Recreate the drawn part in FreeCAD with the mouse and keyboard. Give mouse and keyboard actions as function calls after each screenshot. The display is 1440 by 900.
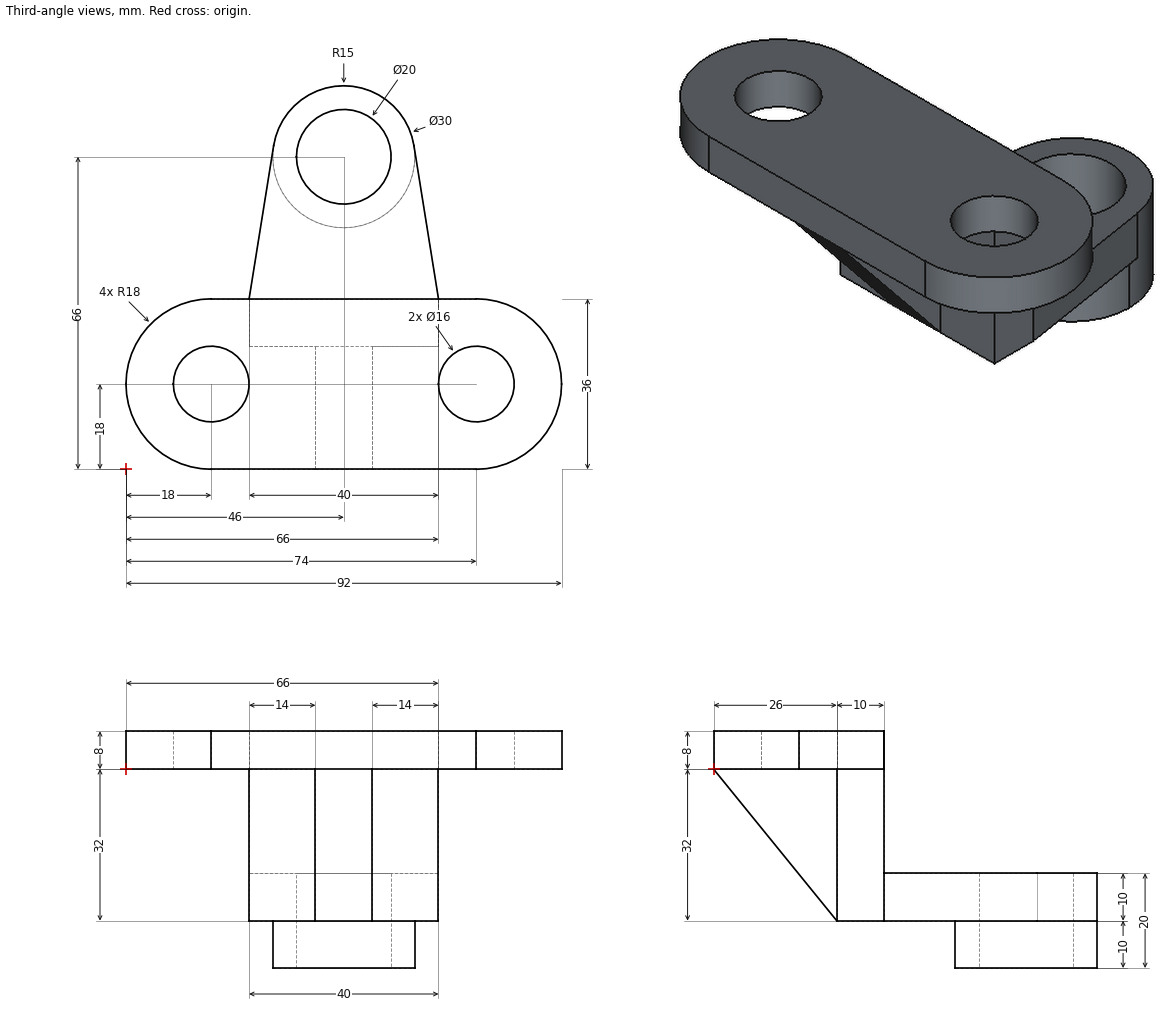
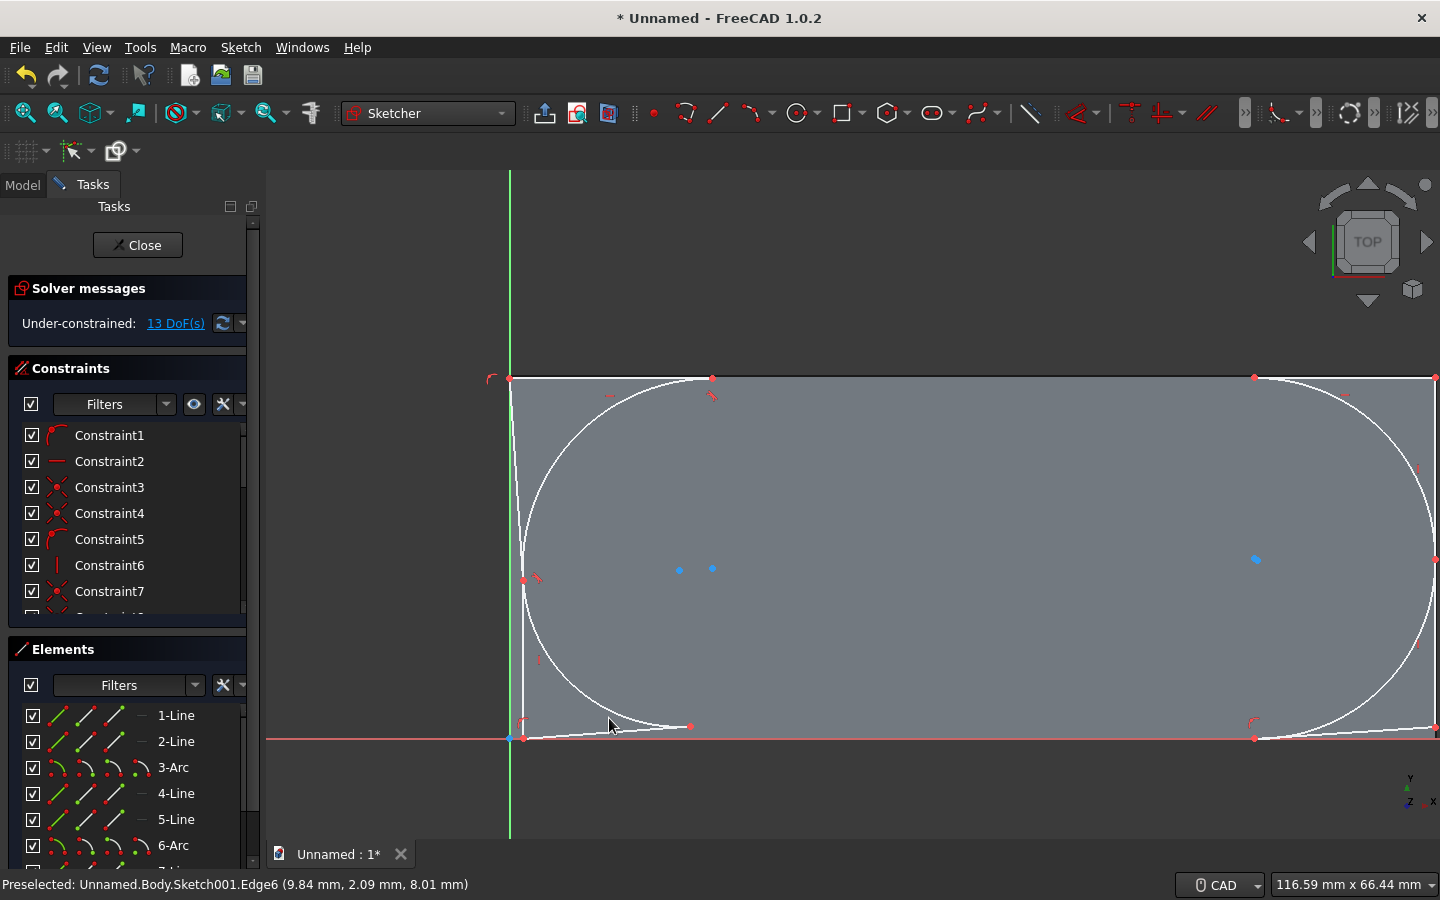
click(573, 735)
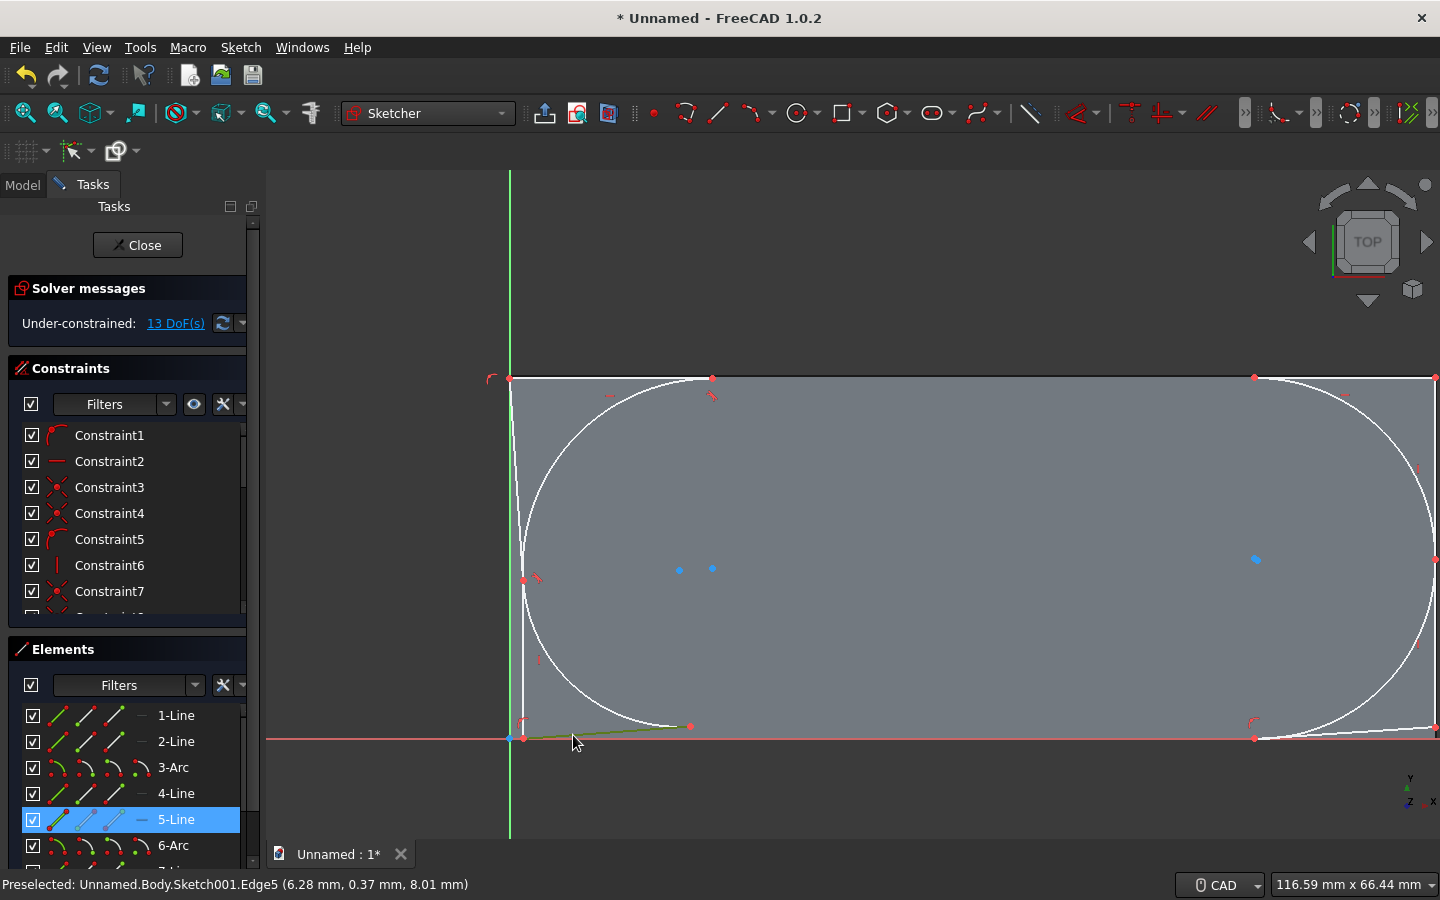
click(545, 651)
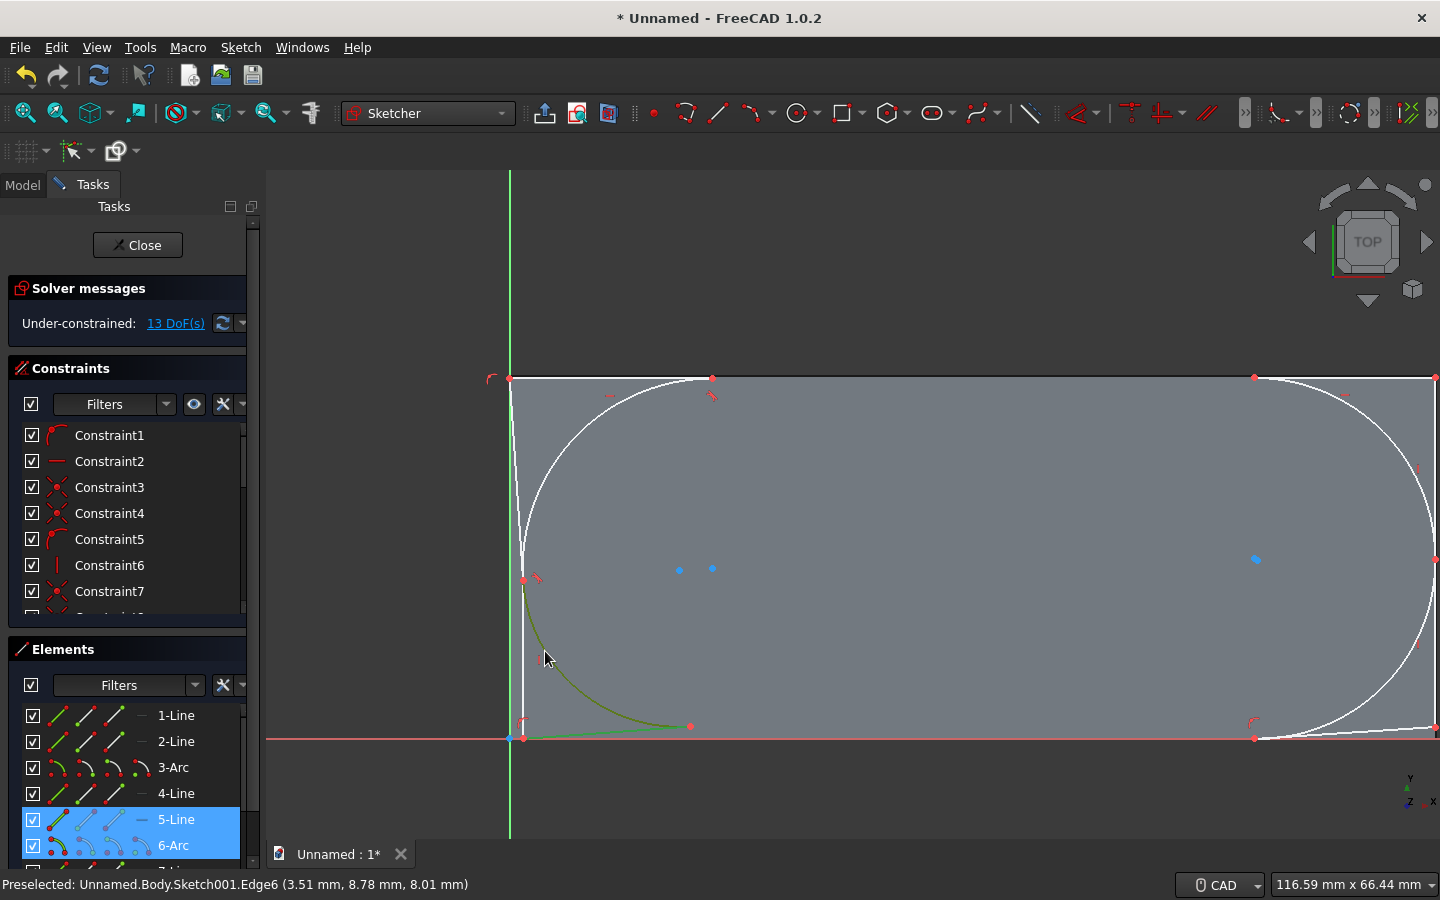
key(t)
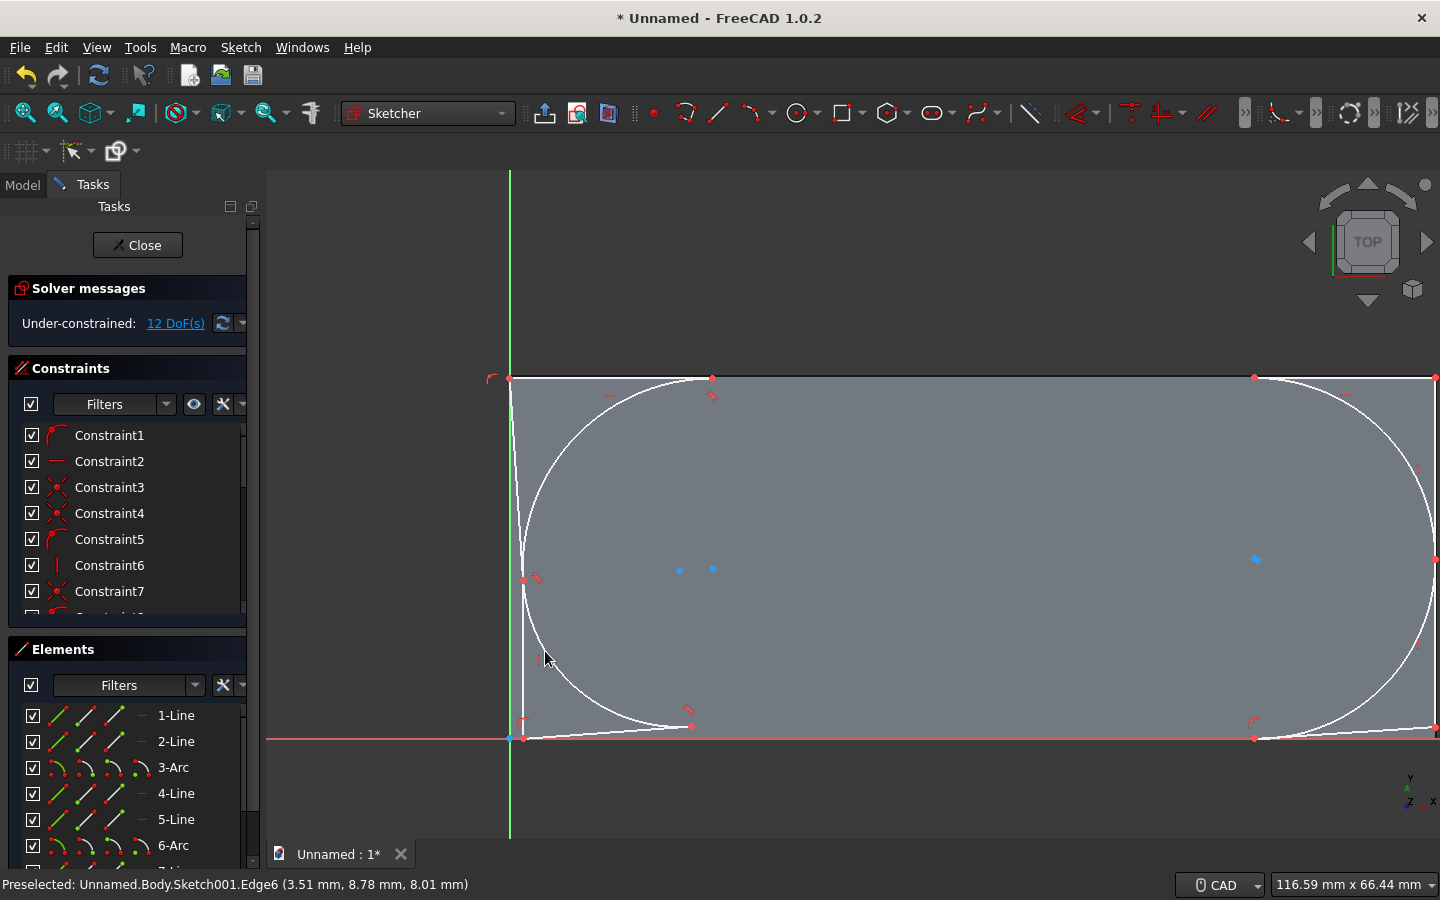
scroll(294, 264, down, 1)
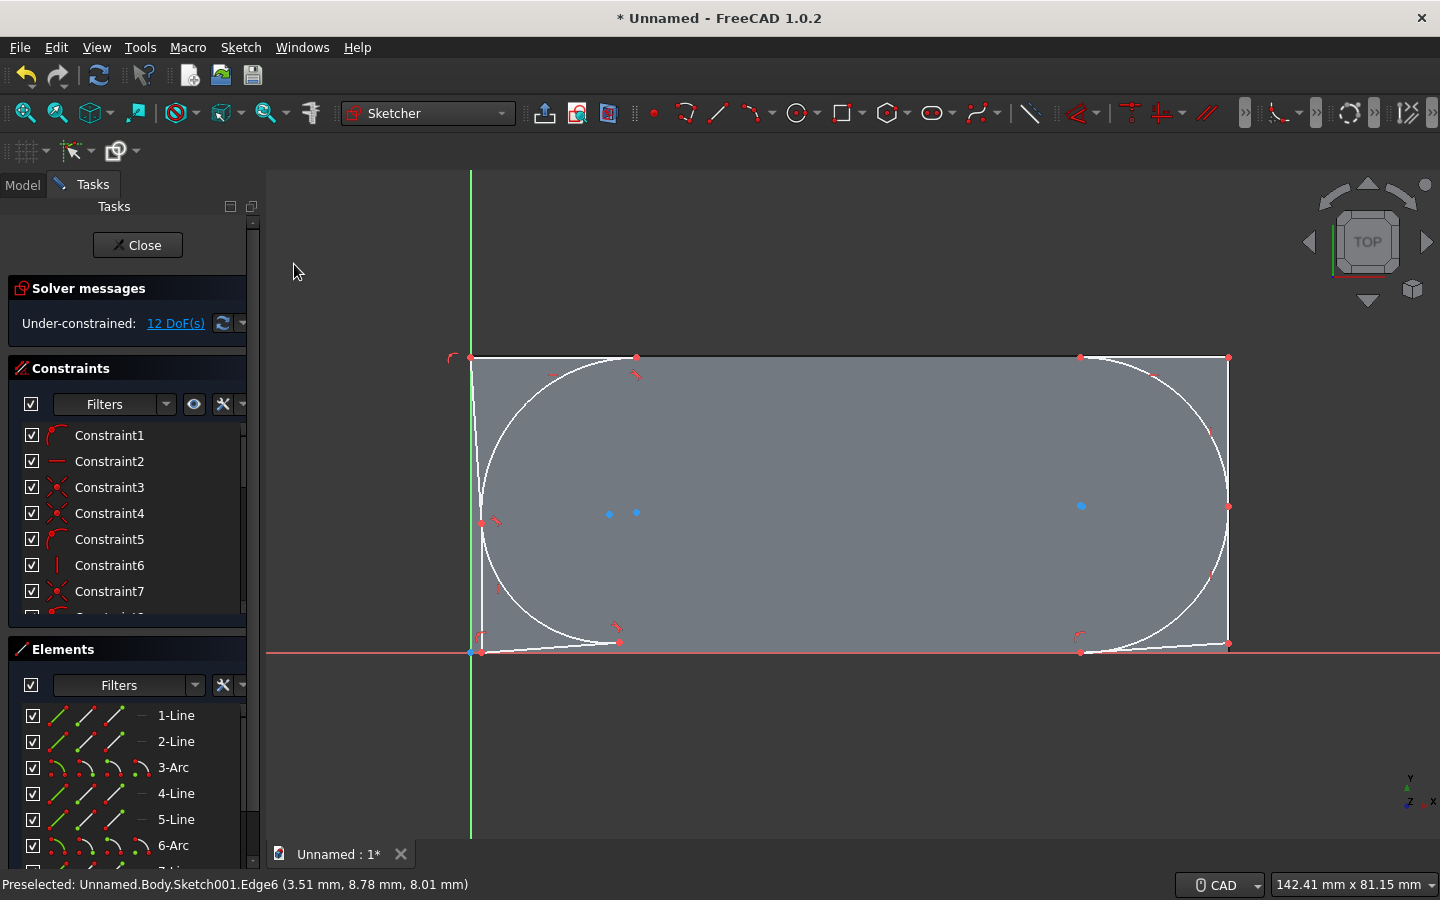
scroll(1199, 645, up, 3)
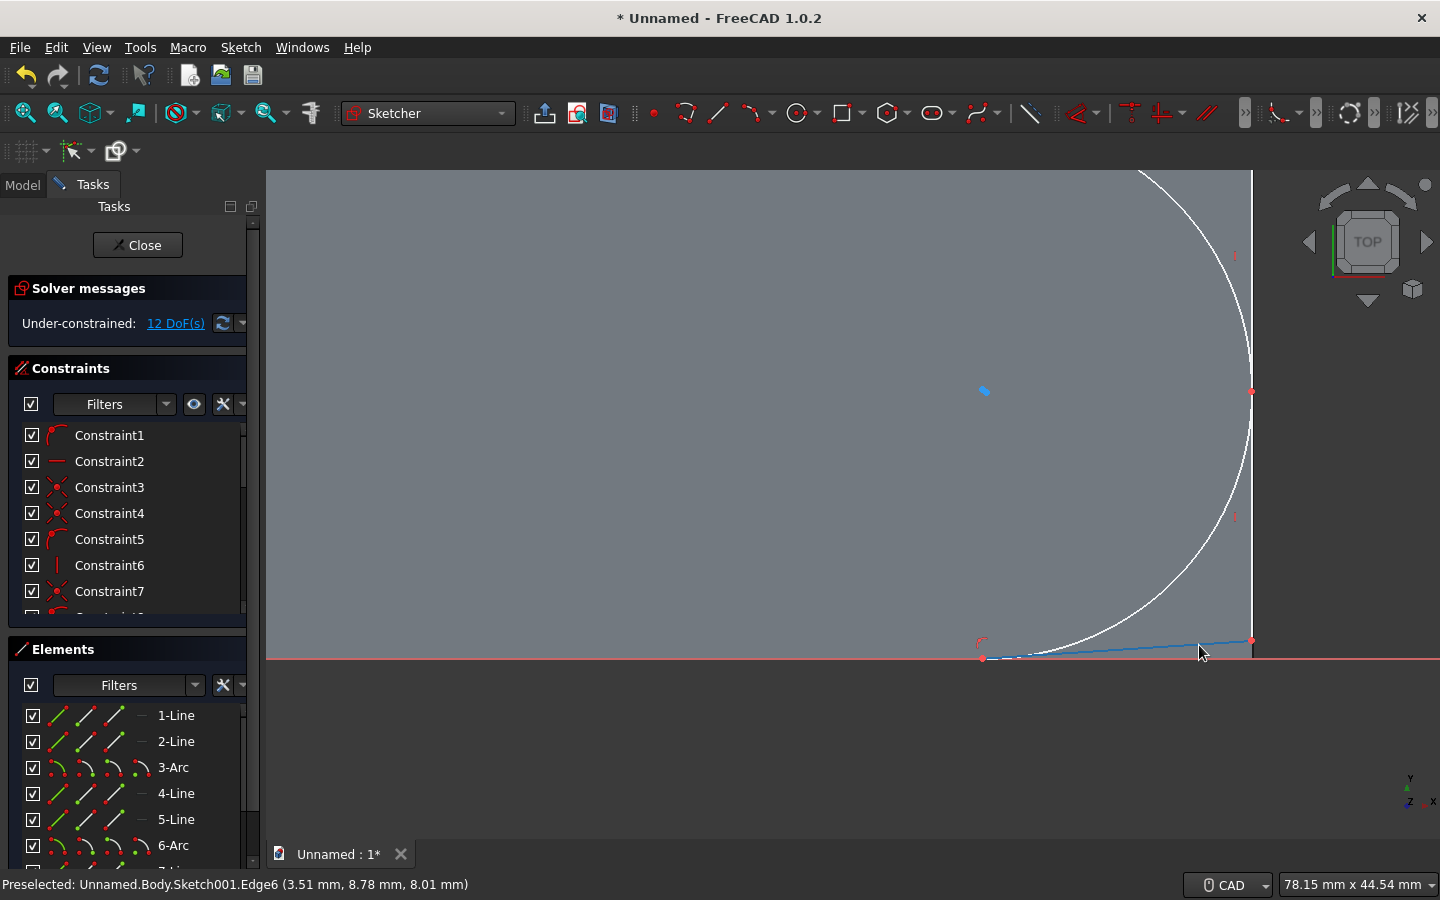
click(1198, 645)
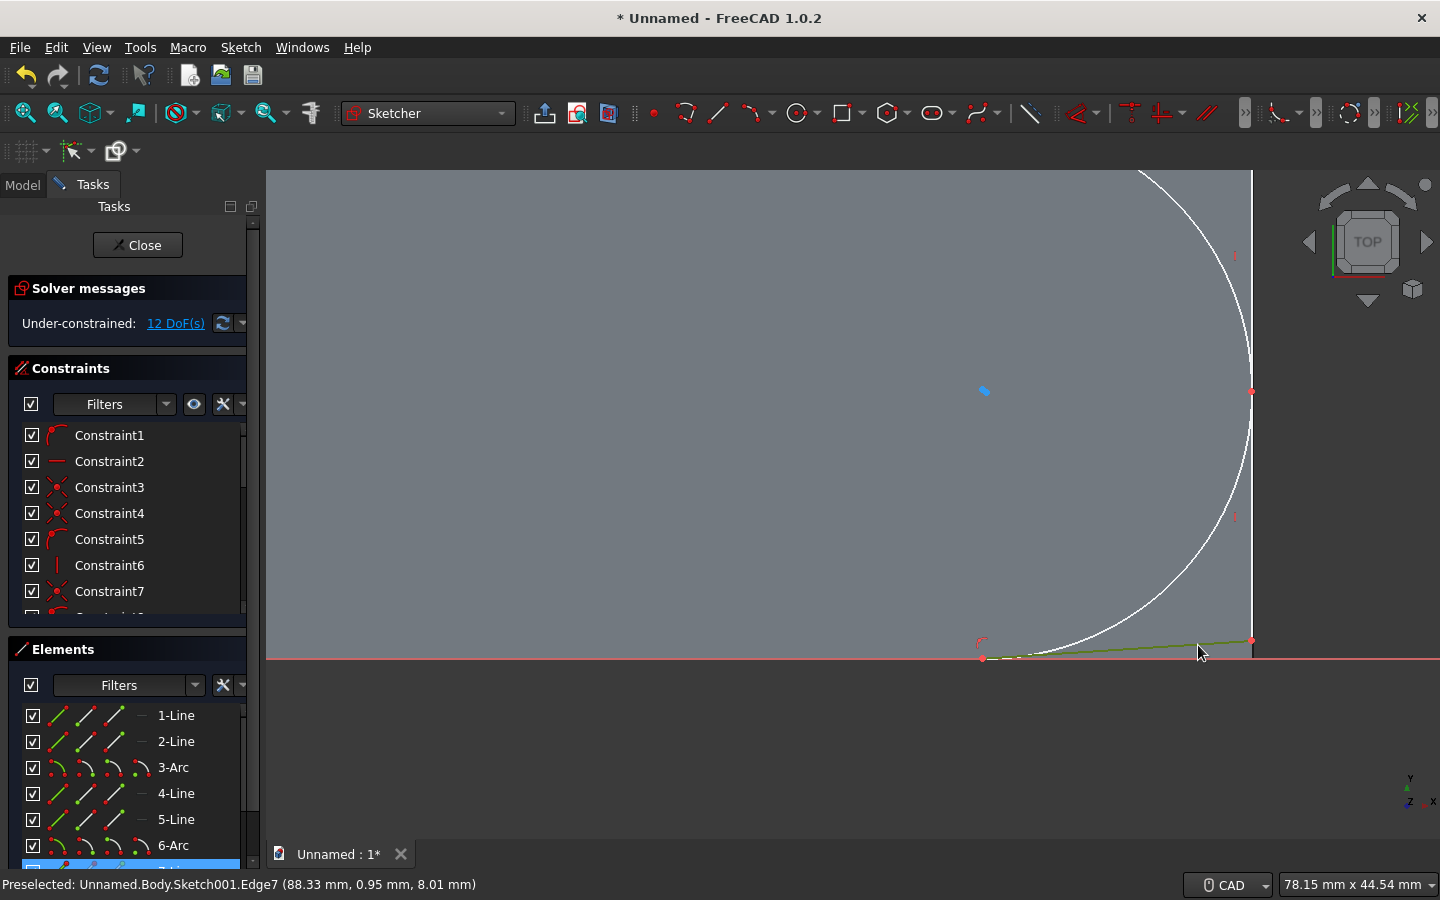
click(1105, 631)